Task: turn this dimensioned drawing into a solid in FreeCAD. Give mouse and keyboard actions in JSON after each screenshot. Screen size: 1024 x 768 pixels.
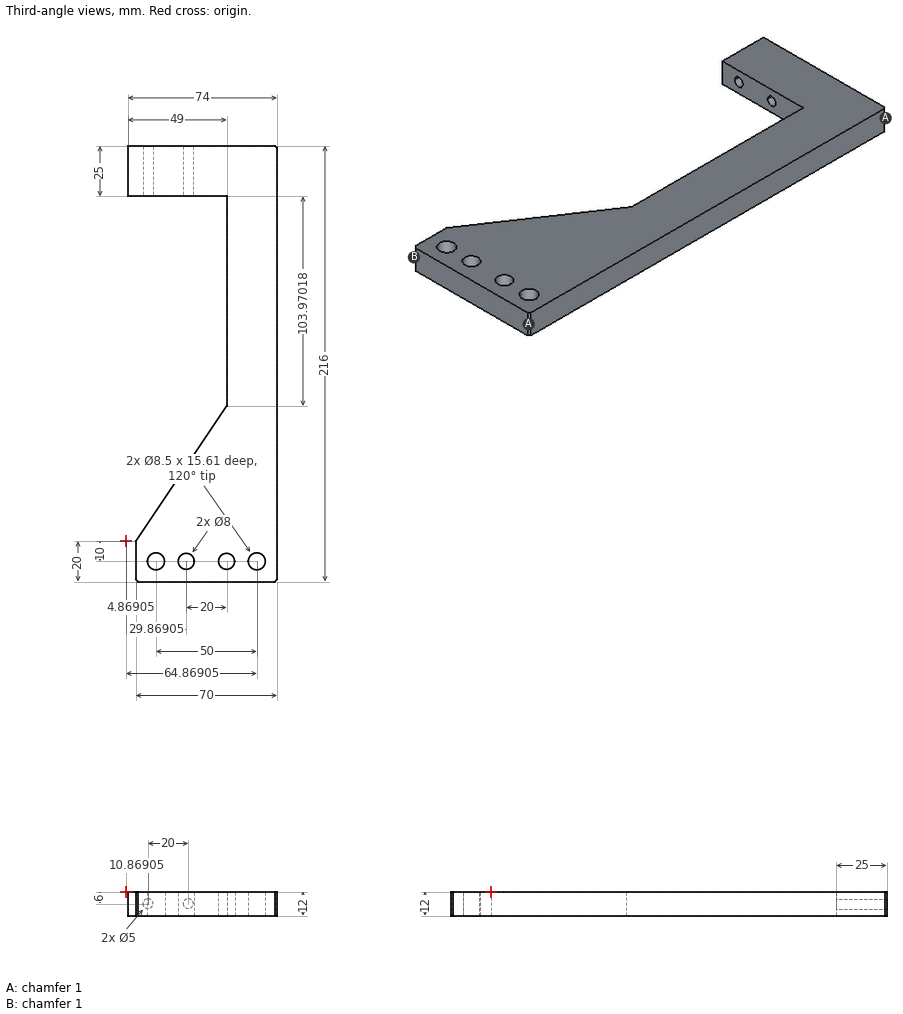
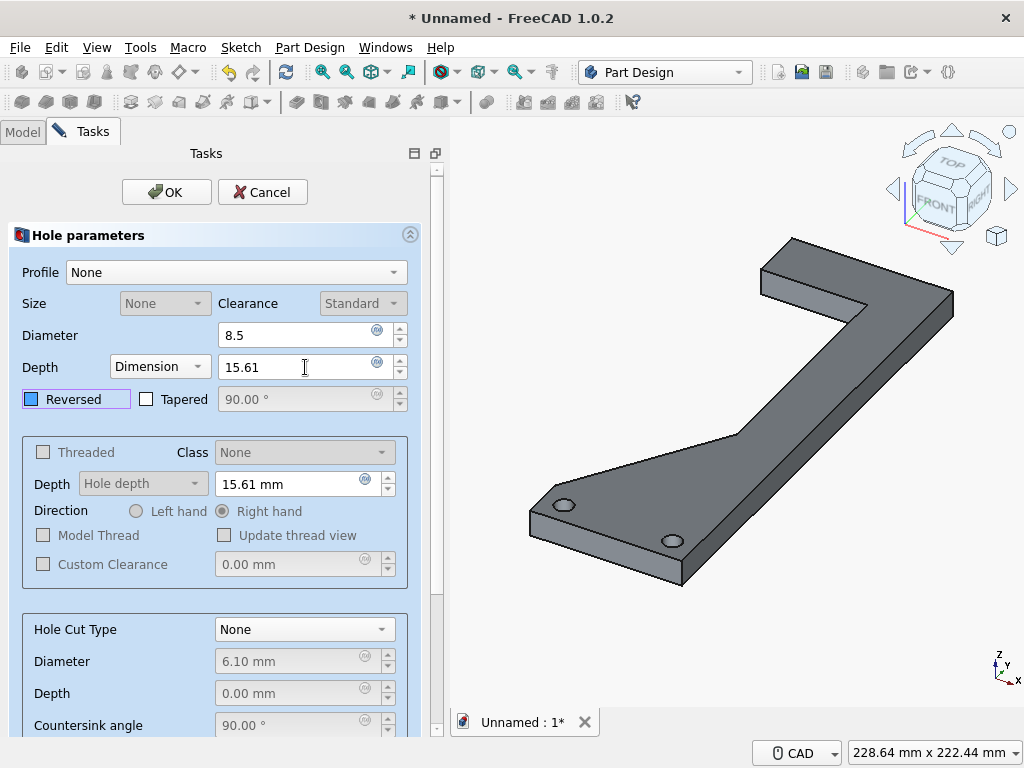
{"action": "scroll", "coordinate": [437, 450], "scroll_direction": "down", "scroll_amount": 3}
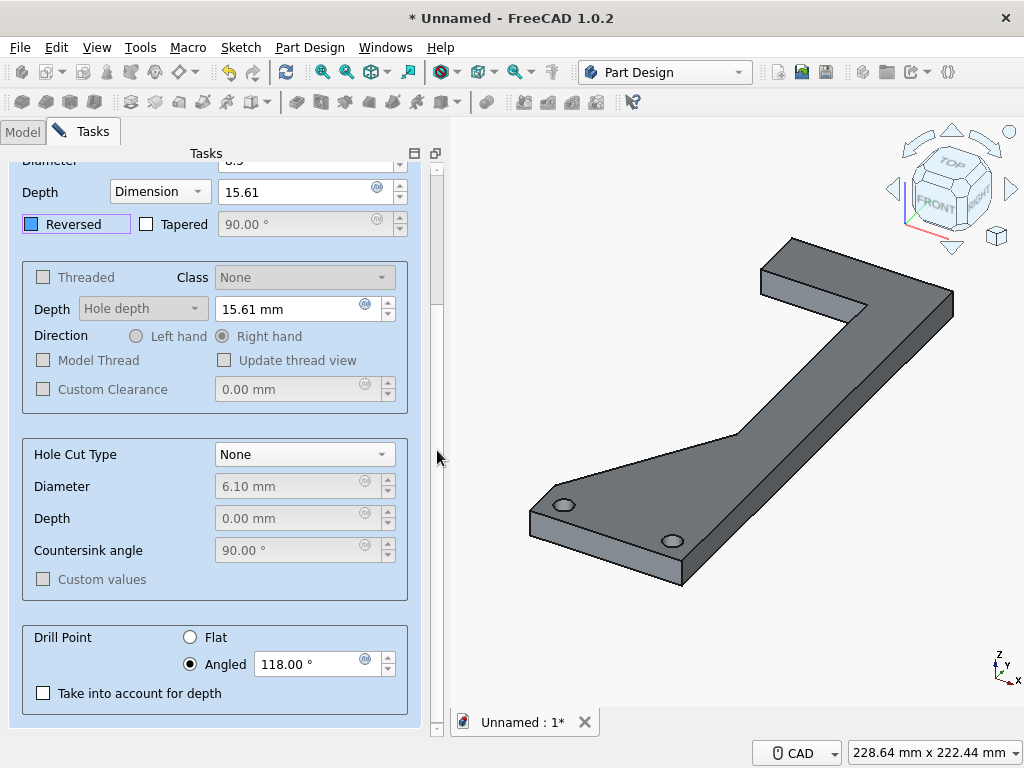
{"action": "triple_click", "coordinate": [317, 664]}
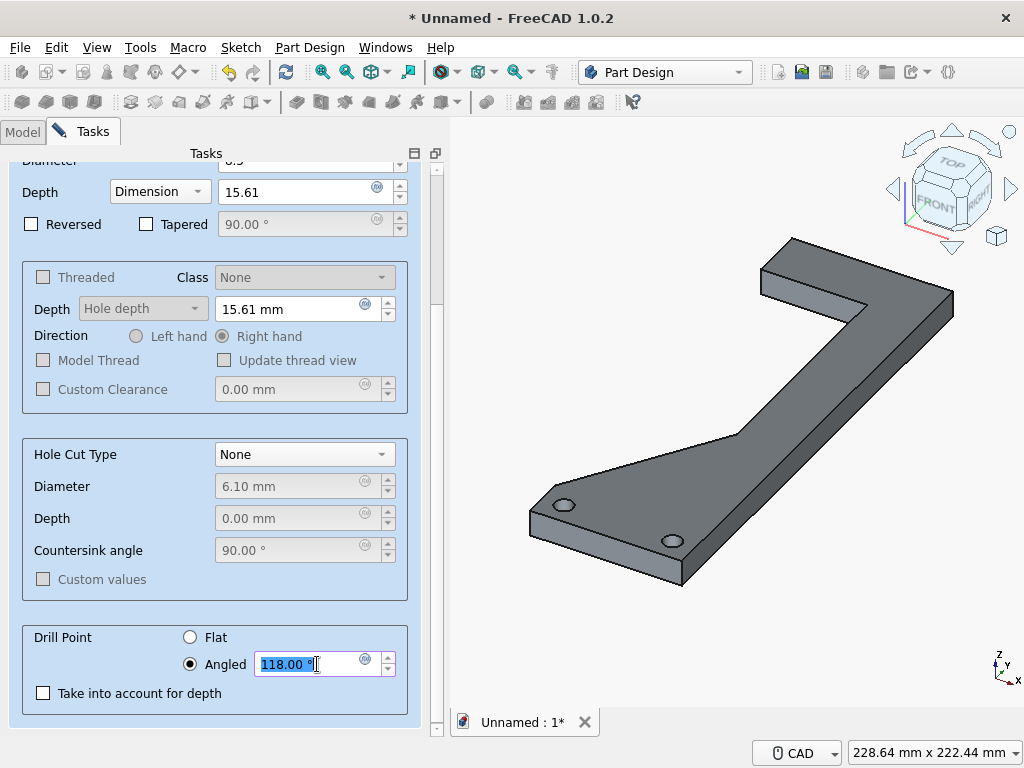
{"action": "type", "text": "120"}
{"action": "key", "text": "Tab"}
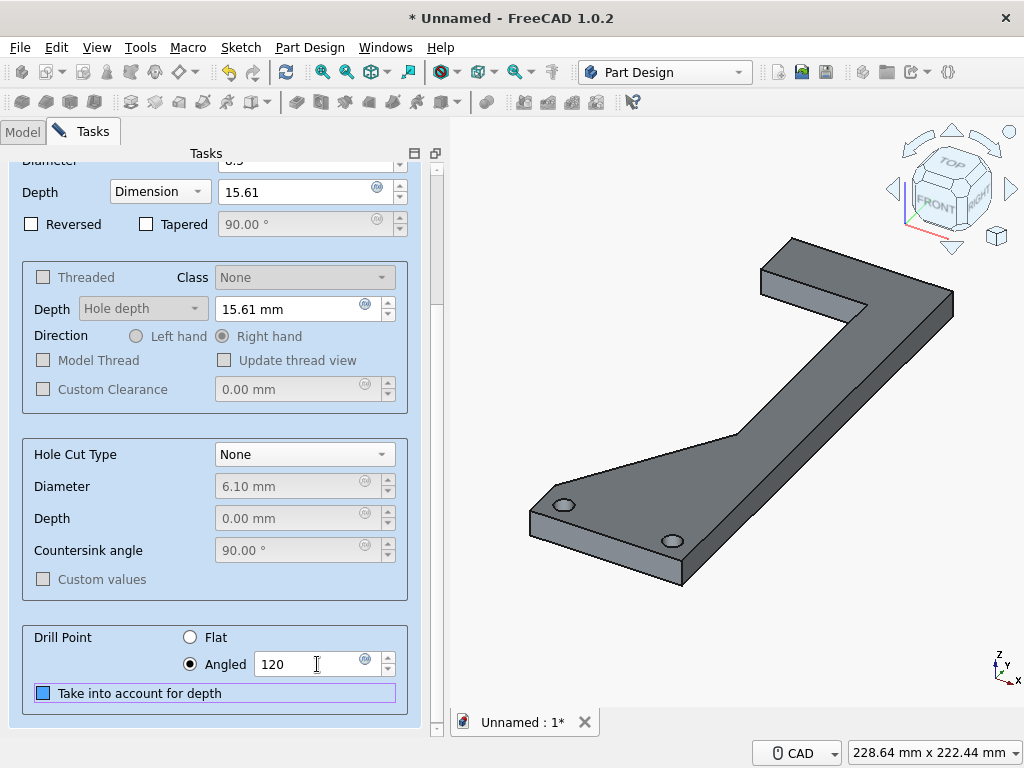
{"action": "scroll", "coordinate": [437, 450], "scroll_direction": "up", "scroll_amount": 4}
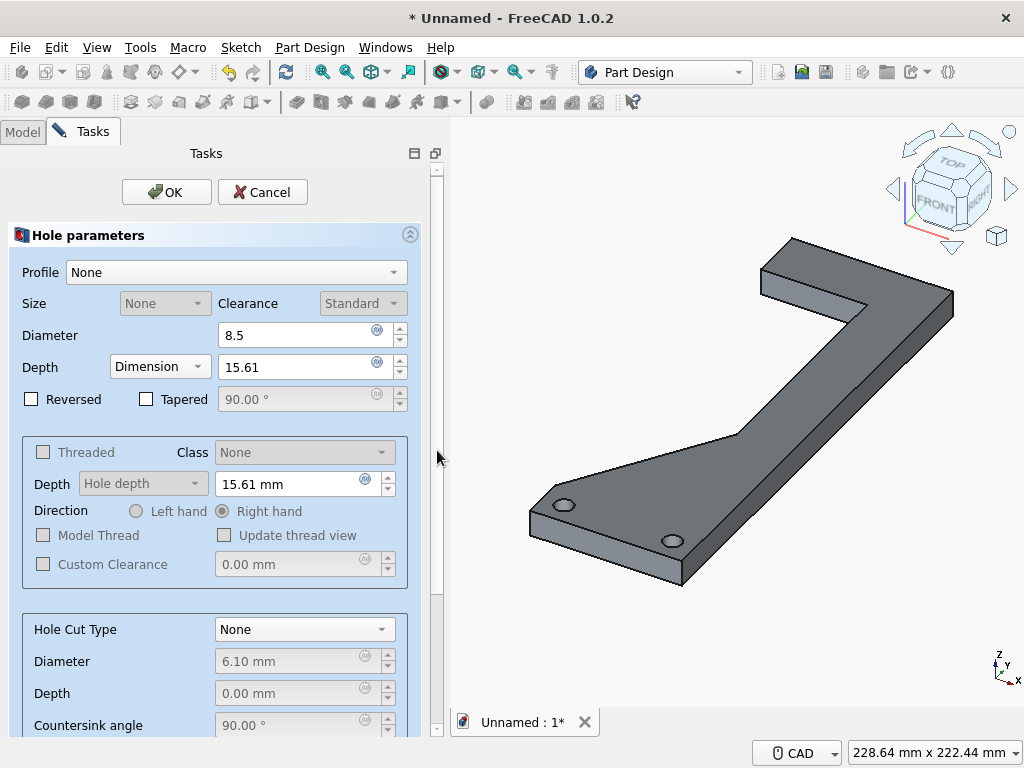
{"action": "left_click", "coordinate": [167, 192]}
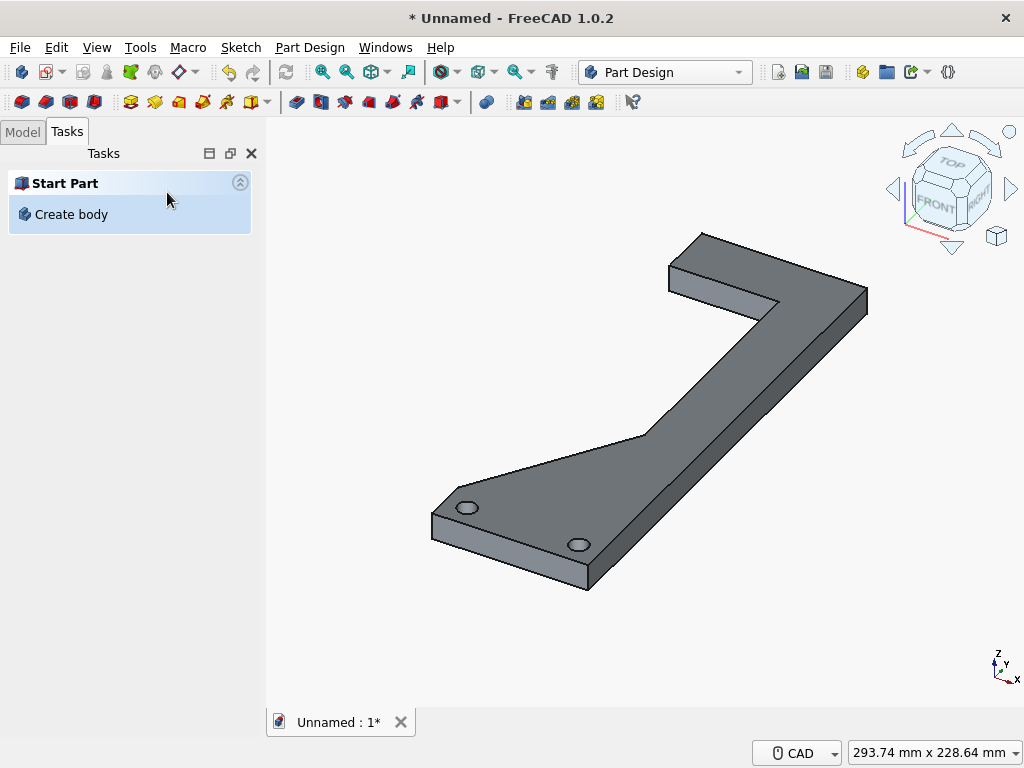
{"action": "left_click", "coordinate": [589, 485]}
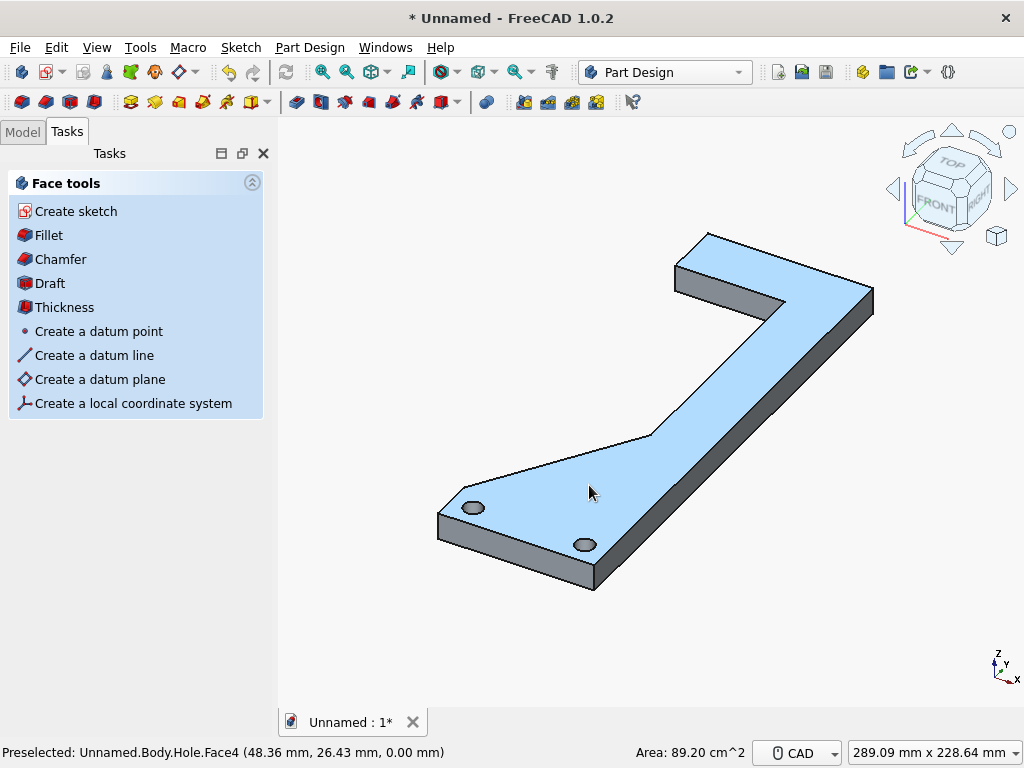
{"action": "left_click", "coordinate": [46, 72]}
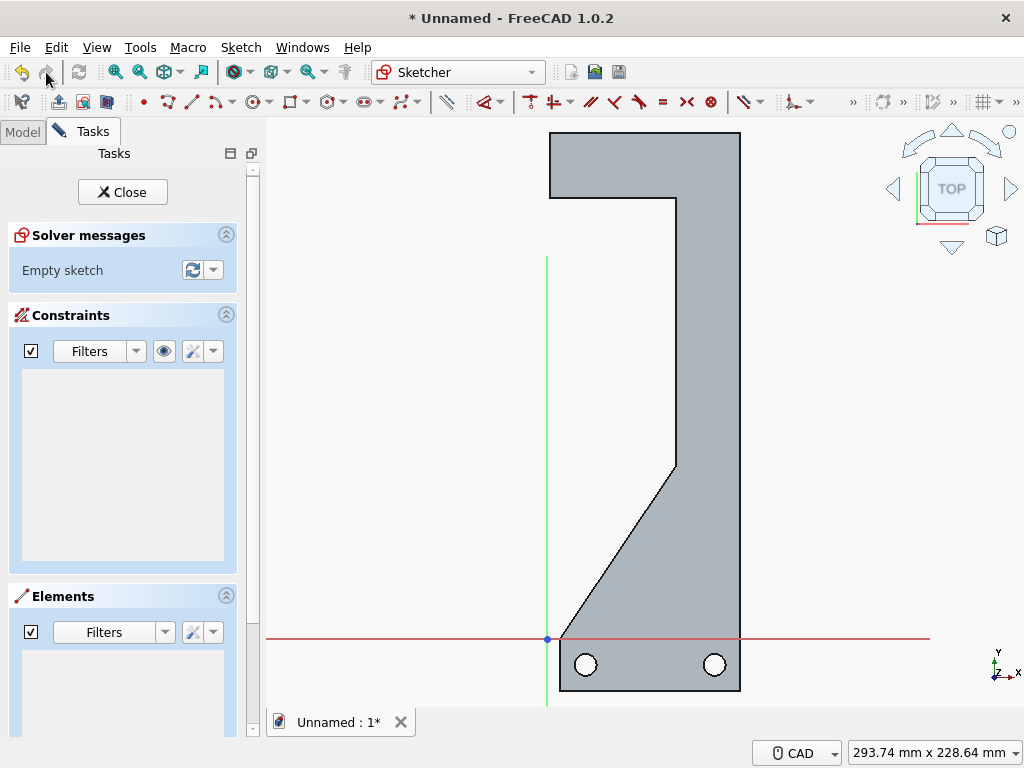
{"action": "scroll", "coordinate": [576, 412], "scroll_direction": "down", "scroll_amount": 5}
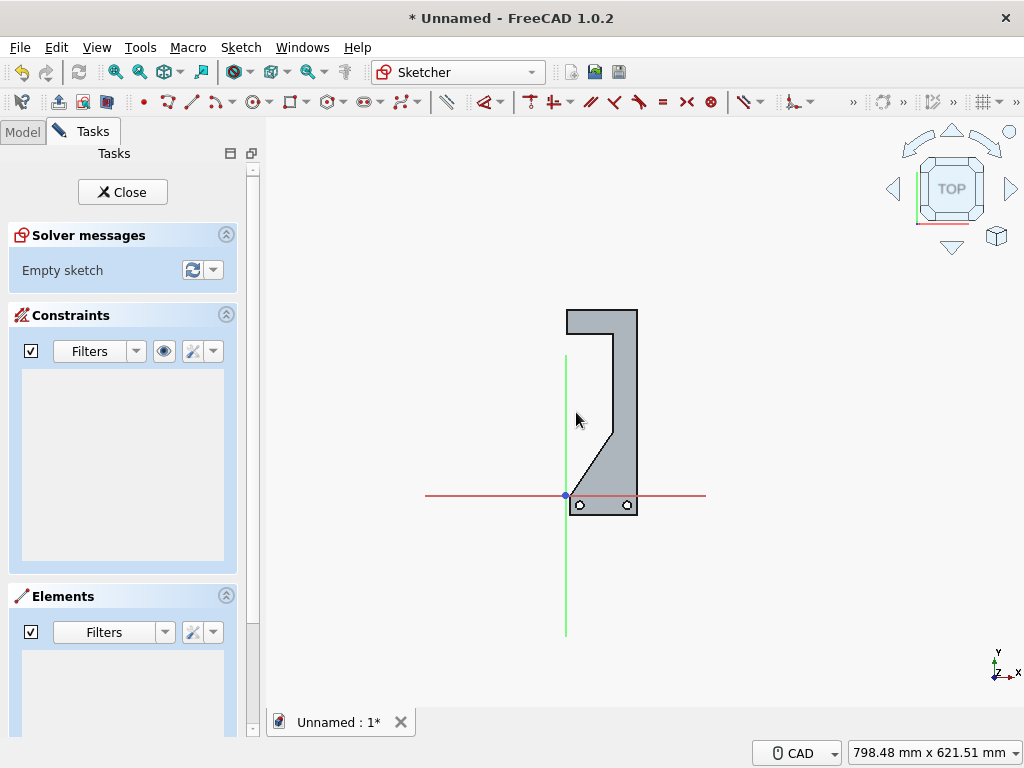
{"action": "scroll", "coordinate": [594, 517], "scroll_direction": "up", "scroll_amount": 10}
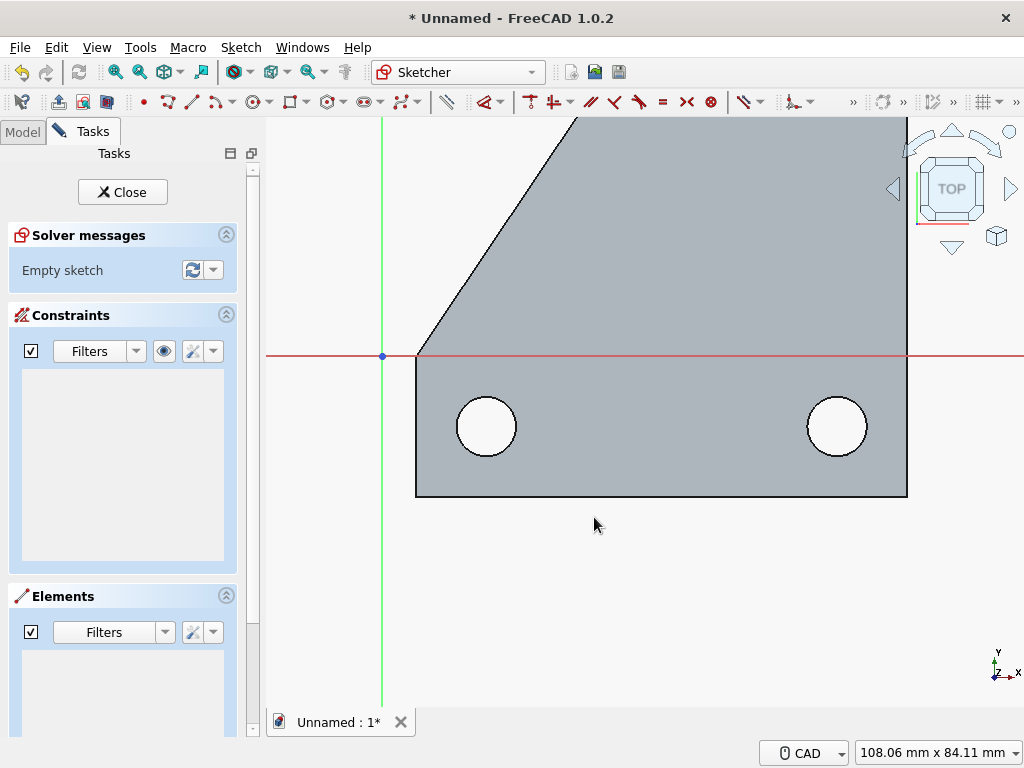
{"action": "left_click", "coordinate": [254, 102]}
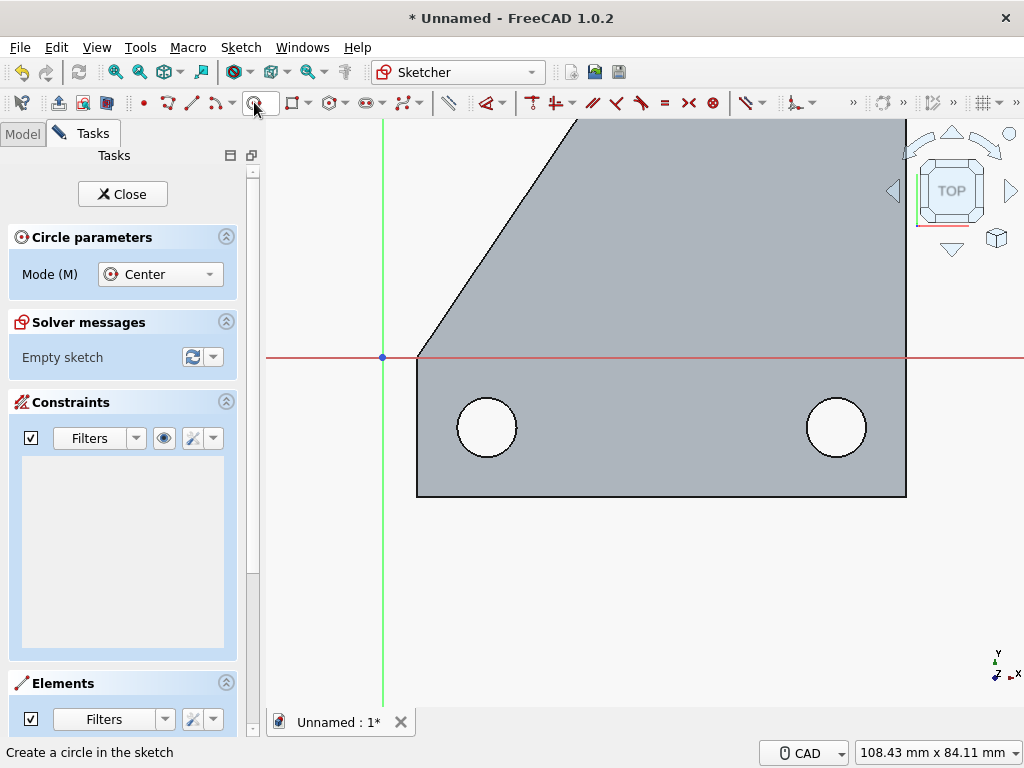
{"action": "left_click", "coordinate": [592, 428]}
{"action": "left_click", "coordinate": [612, 408]}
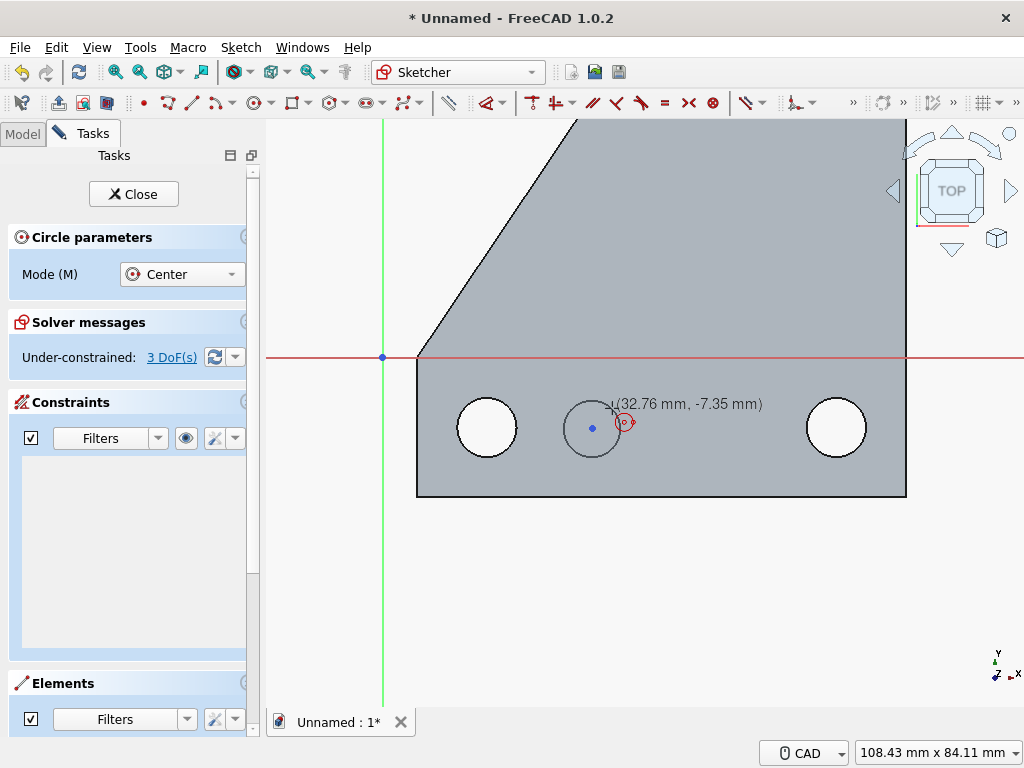
{"action": "left_click", "coordinate": [732, 428]}
{"action": "left_click", "coordinate": [751, 408]}
{"action": "key", "text": "Escape"}